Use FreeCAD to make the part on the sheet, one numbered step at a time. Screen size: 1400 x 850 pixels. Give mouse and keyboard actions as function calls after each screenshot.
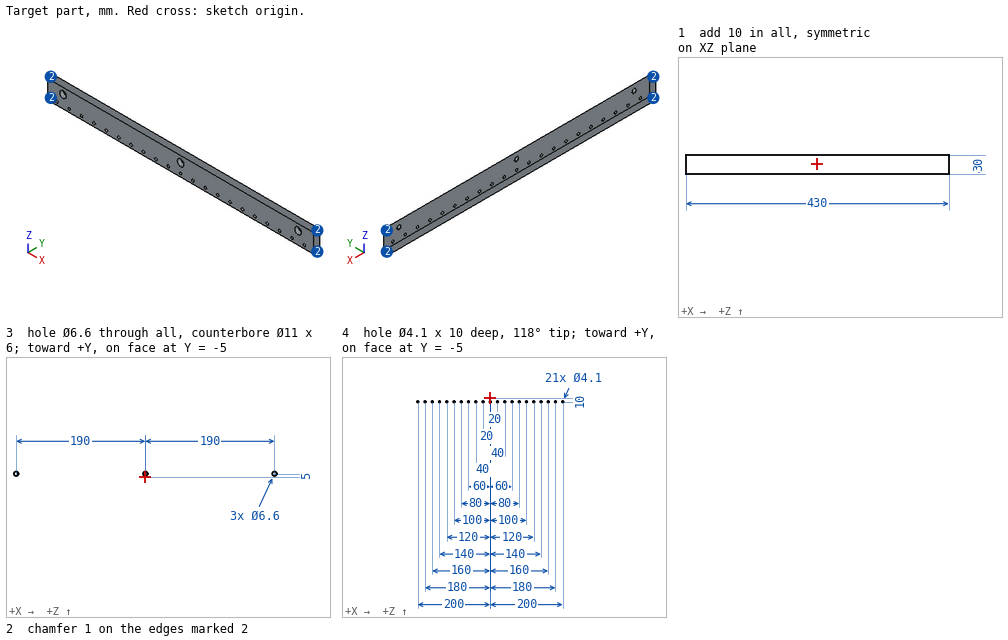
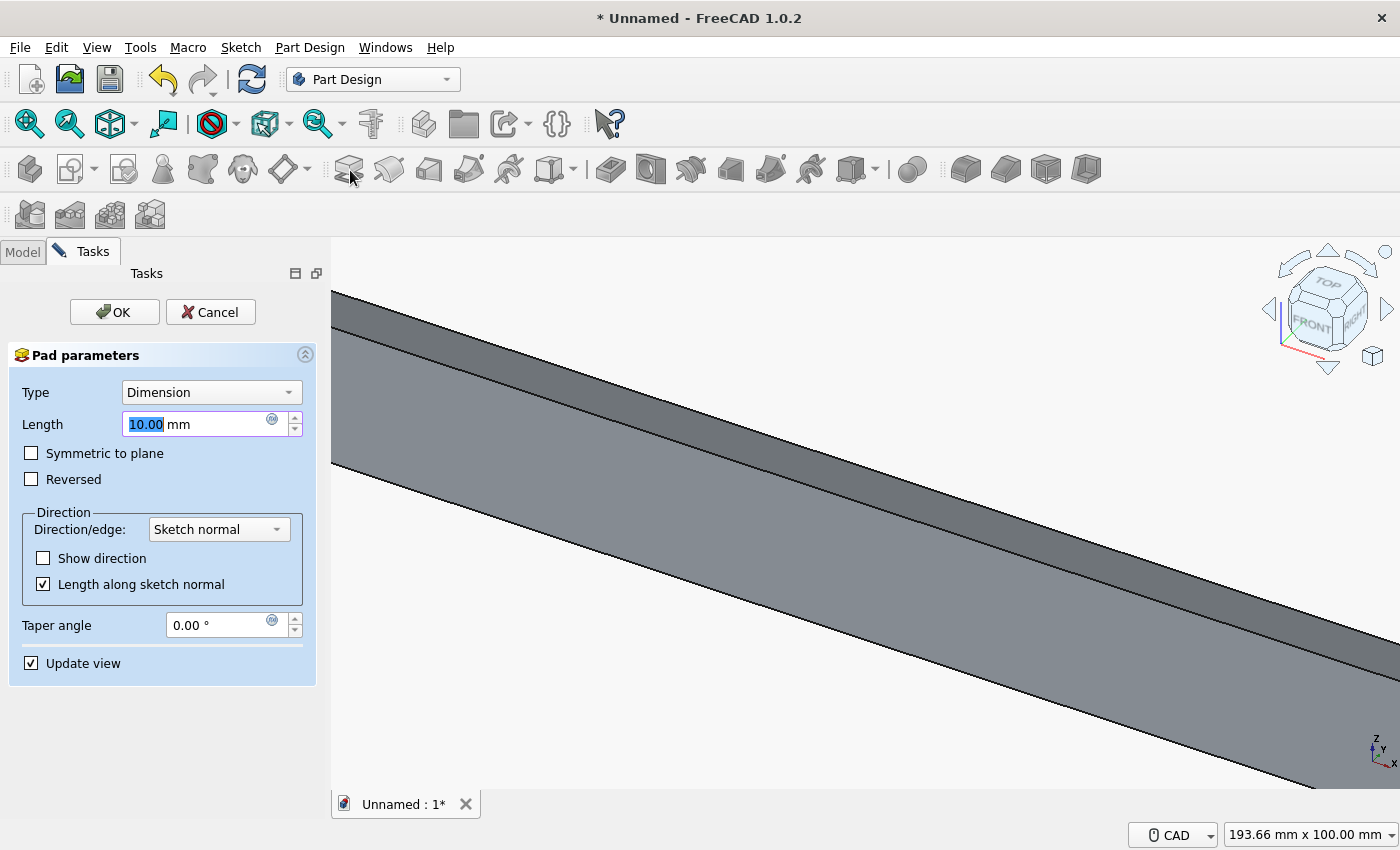
text(10)
key(Tab)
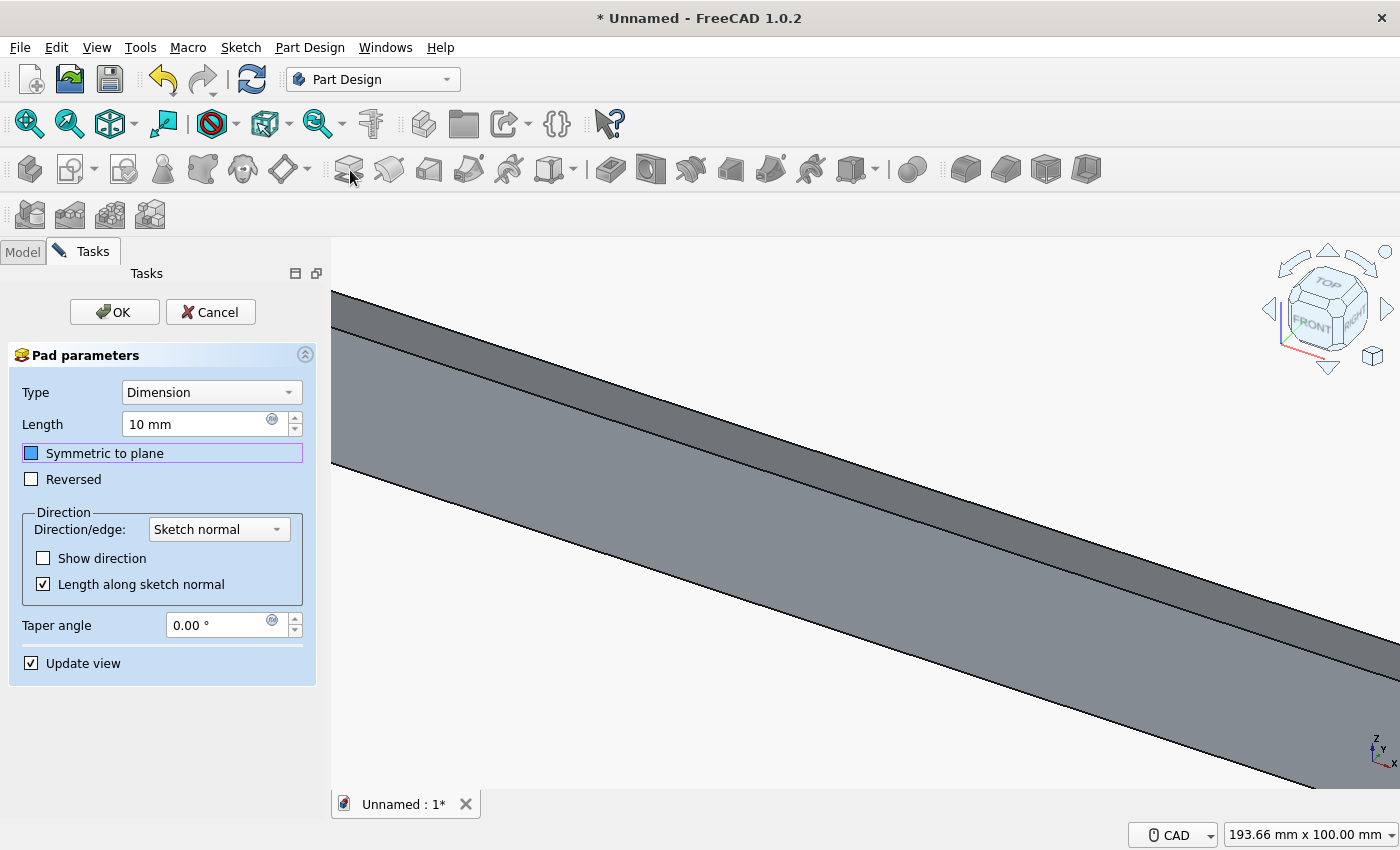
click(30, 453)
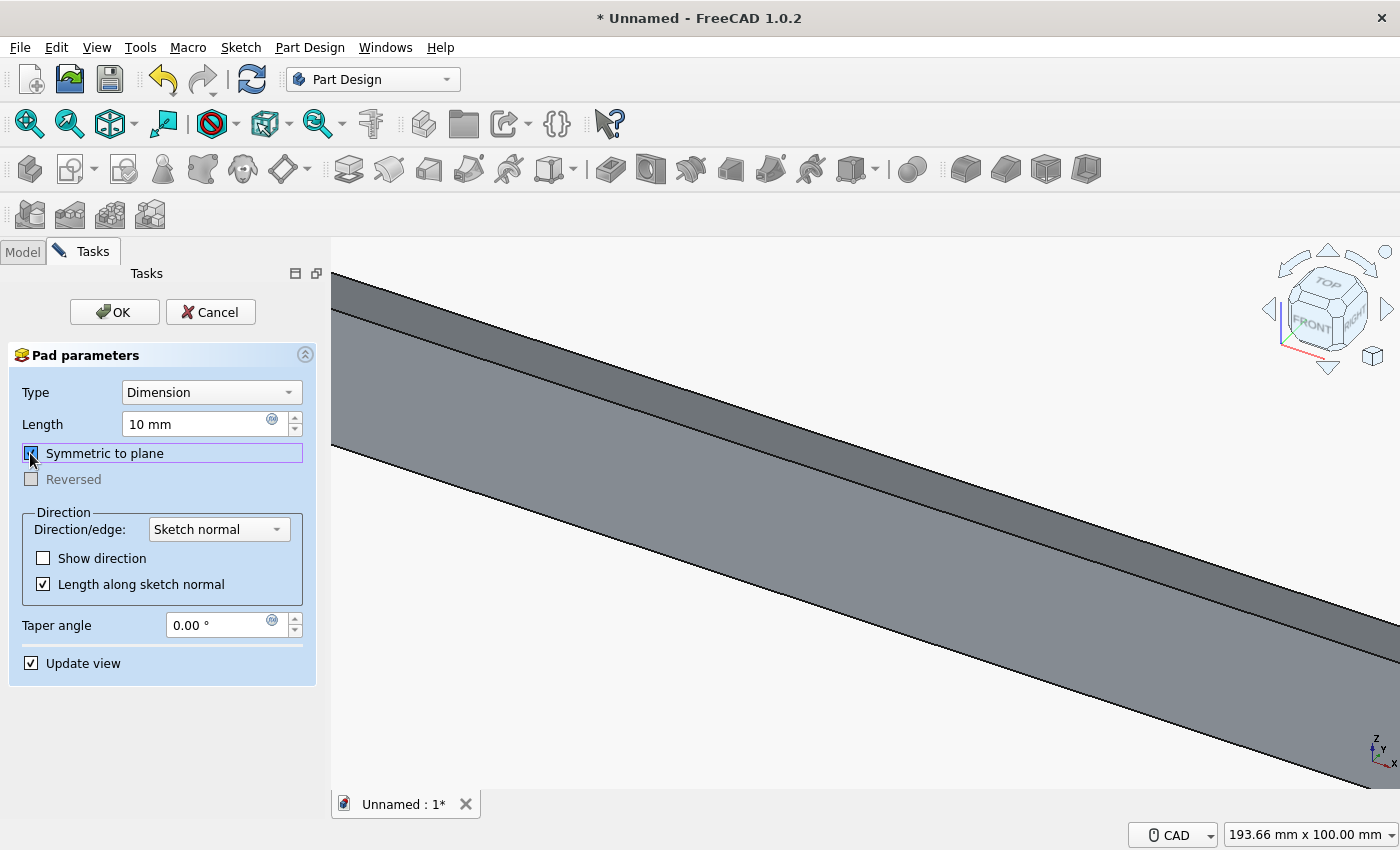
click(115, 312)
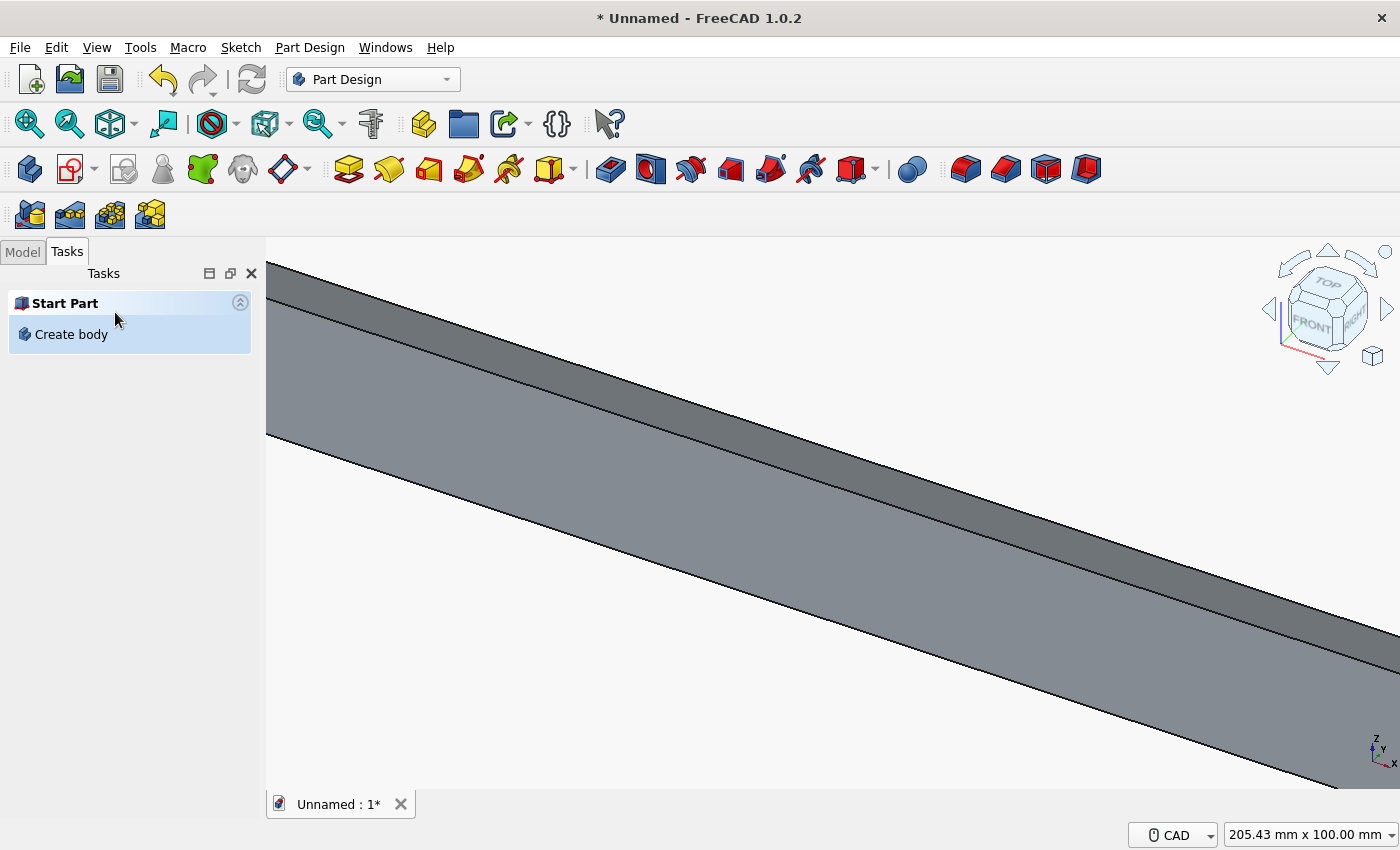
click(30, 124)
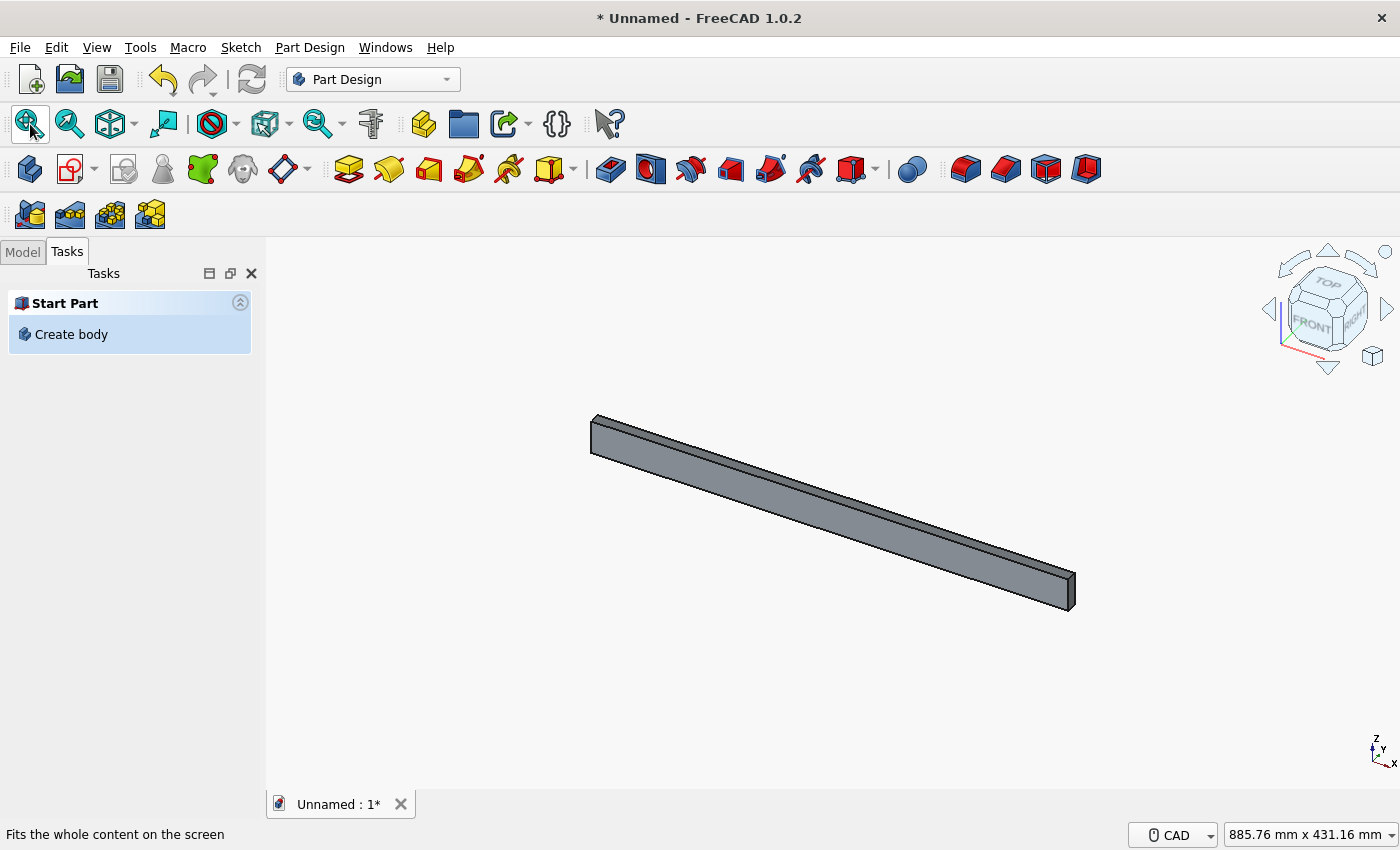
click(1073, 574)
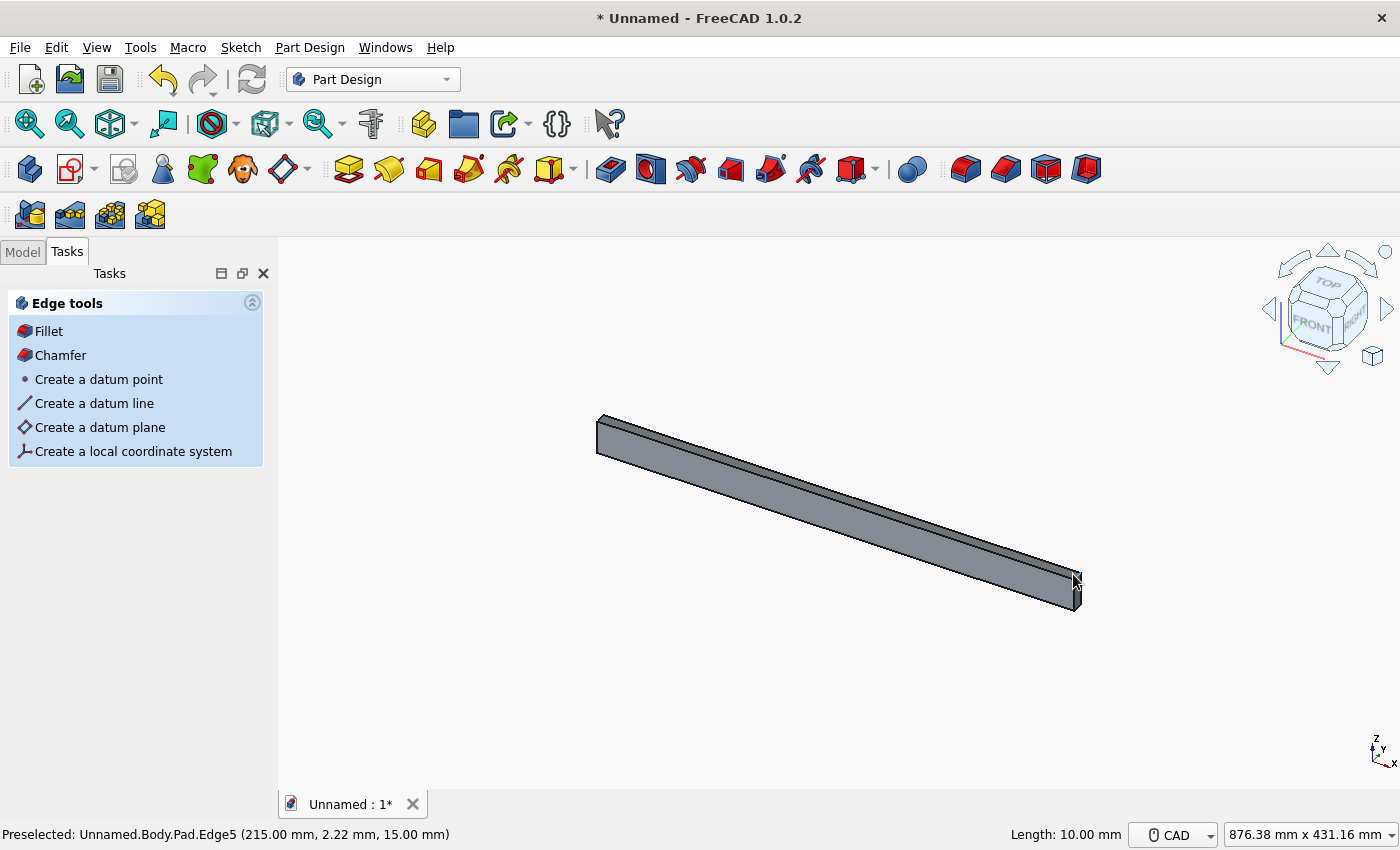
scroll(601, 417, up, 6)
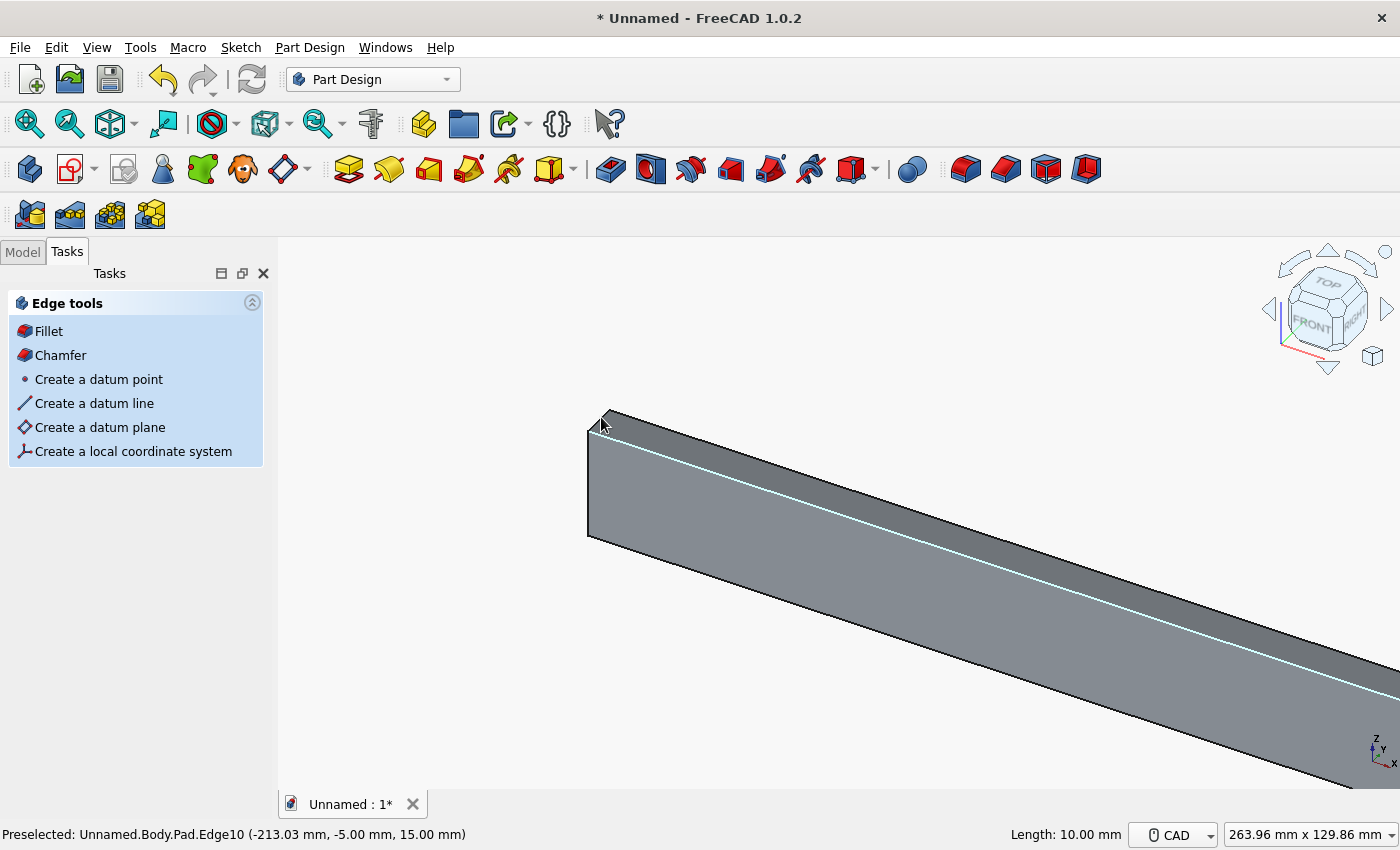
click(30, 124)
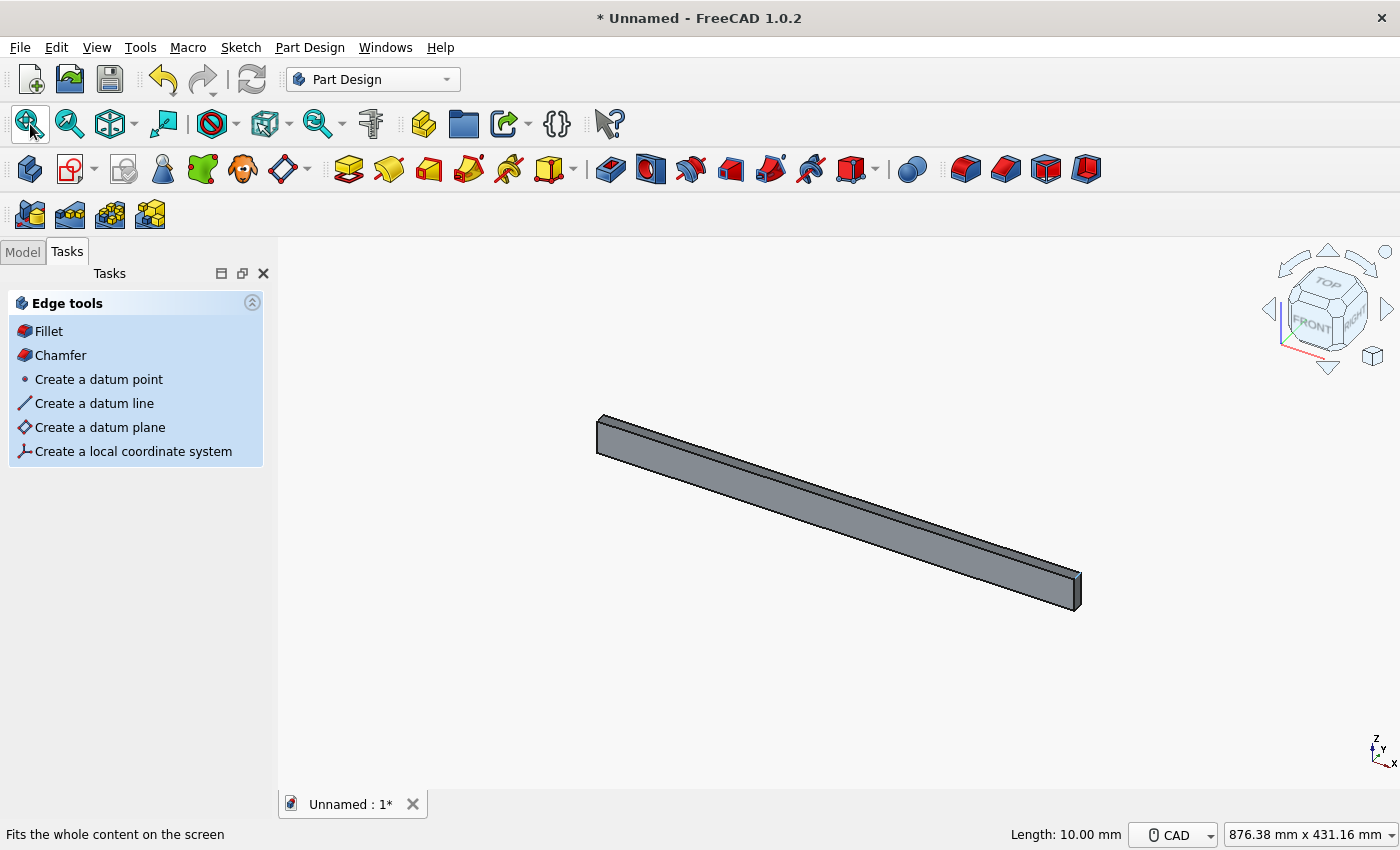
key(0)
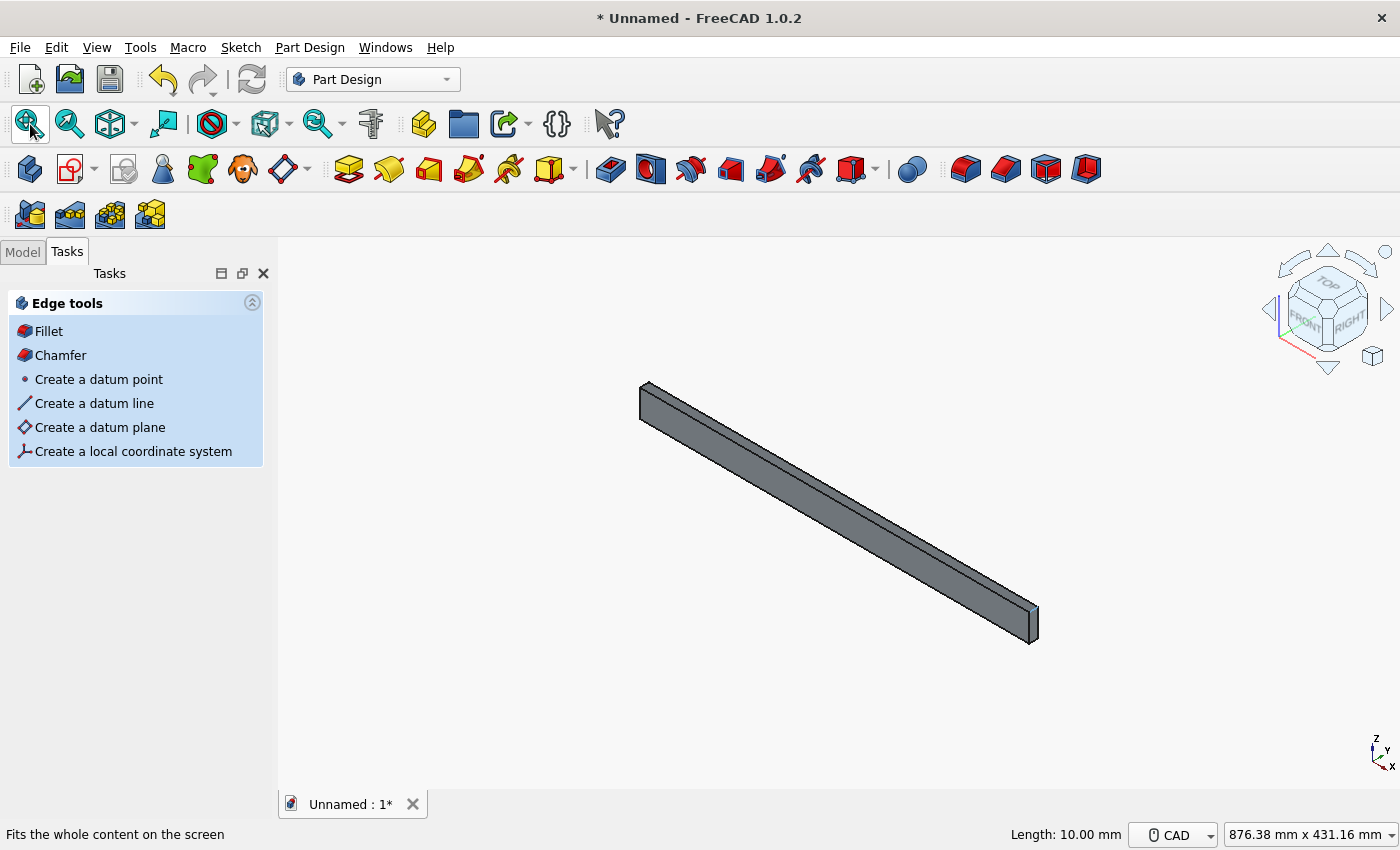
scroll(644, 384, up, 6)